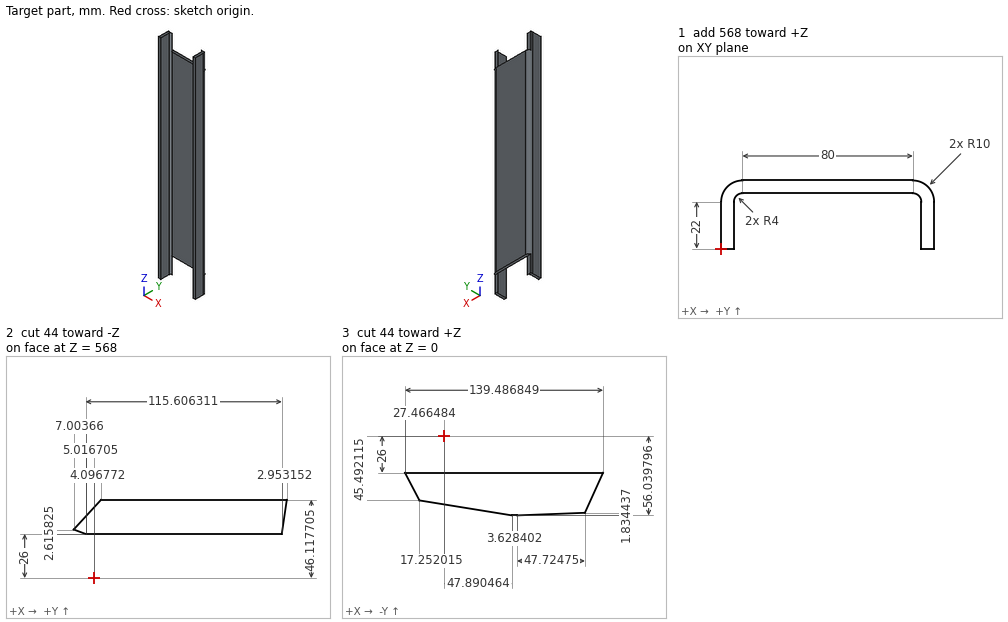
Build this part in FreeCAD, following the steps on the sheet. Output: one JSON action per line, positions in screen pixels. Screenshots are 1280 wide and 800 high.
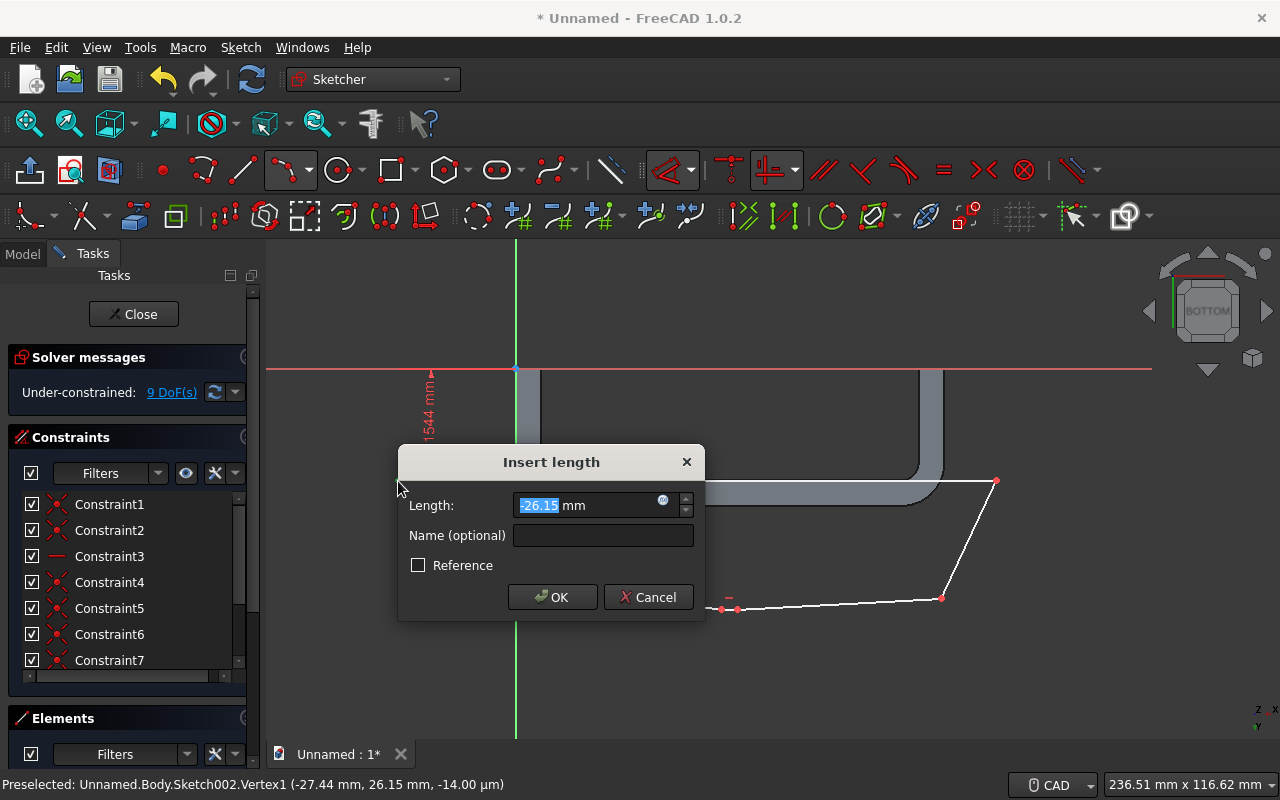
{"action": "type", "text": "-26"}
{"action": "key", "text": "Return"}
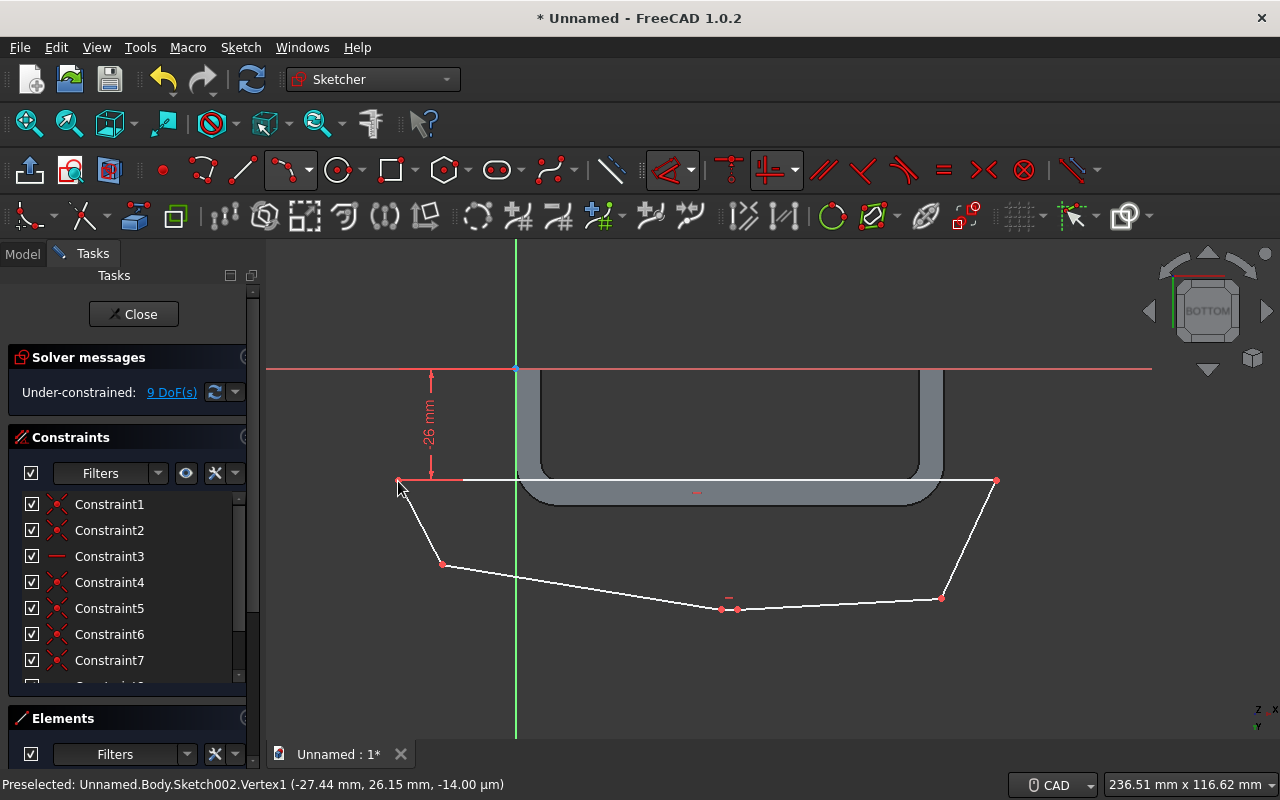
{"action": "scroll", "coordinate": [729, 610], "scroll_direction": "up", "scroll_amount": 5}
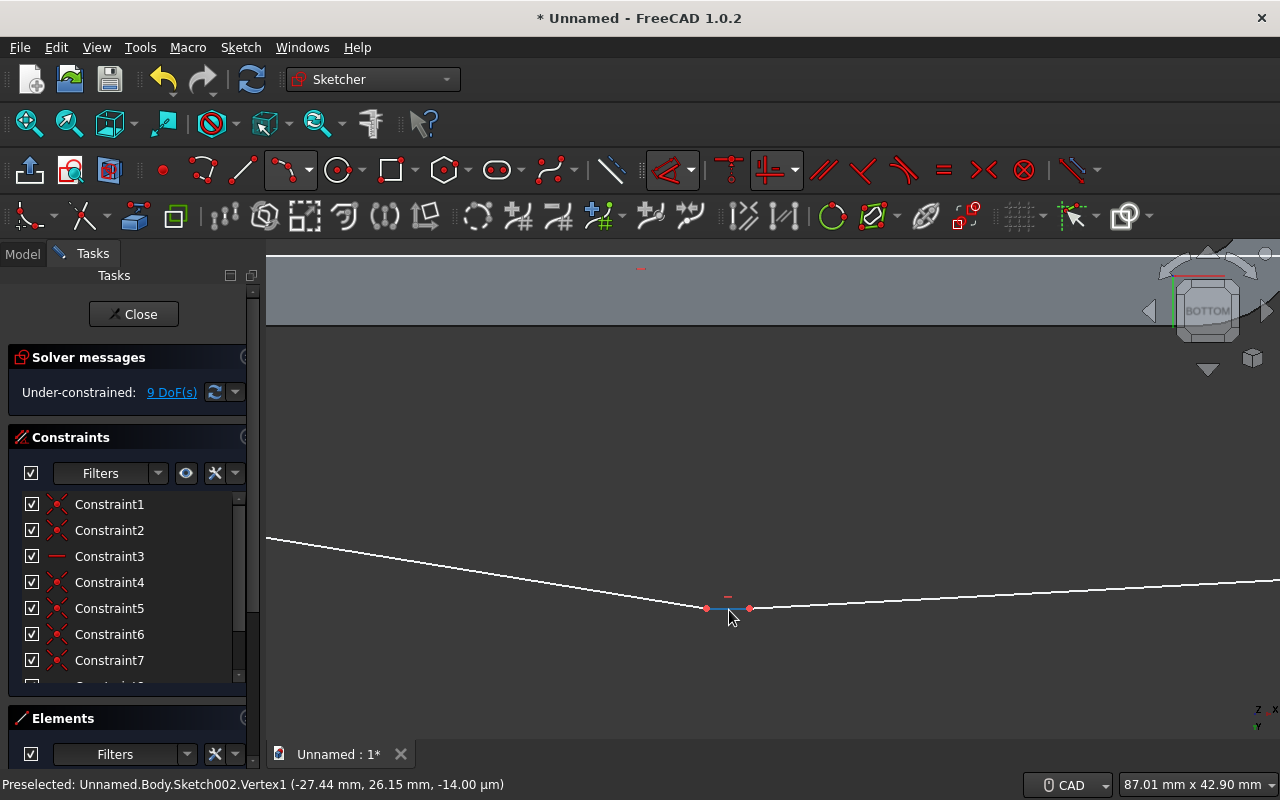
{"action": "left_click", "coordinate": [728, 609]}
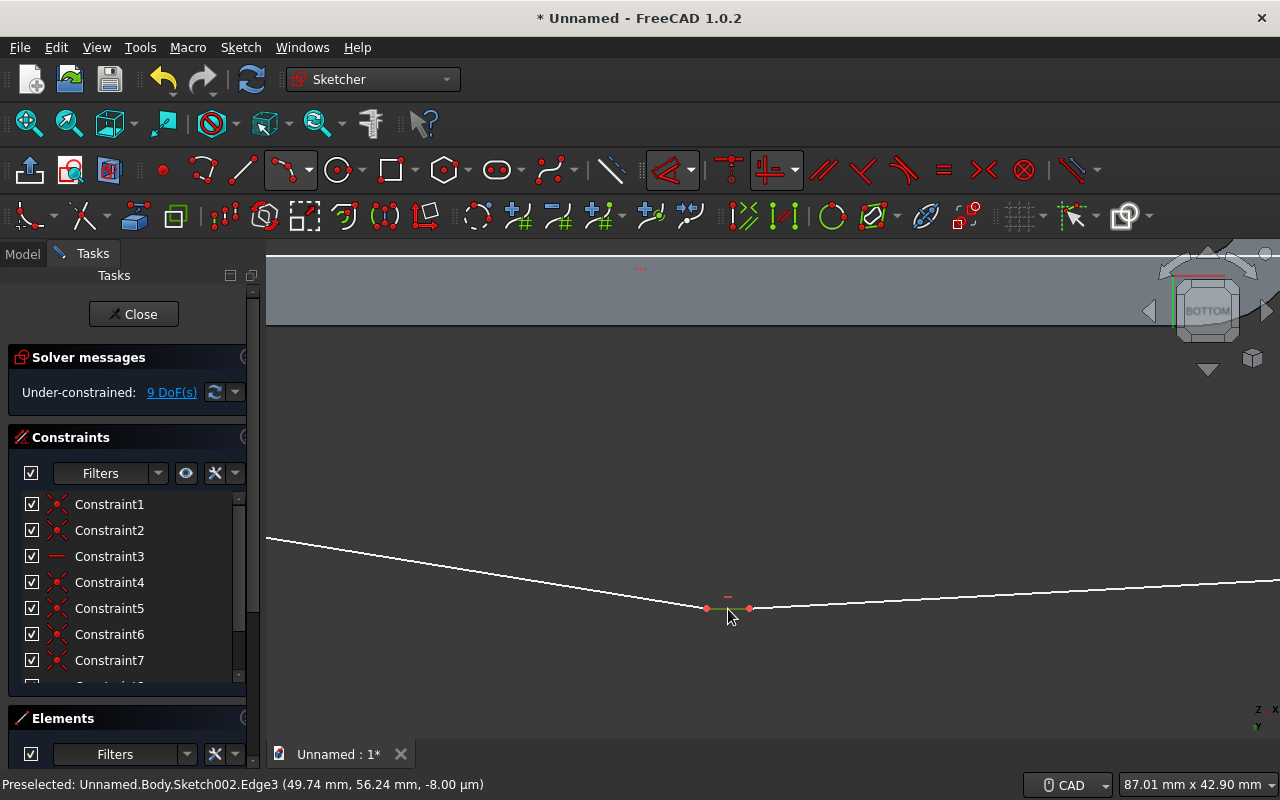
{"action": "left_click", "coordinate": [694, 170]}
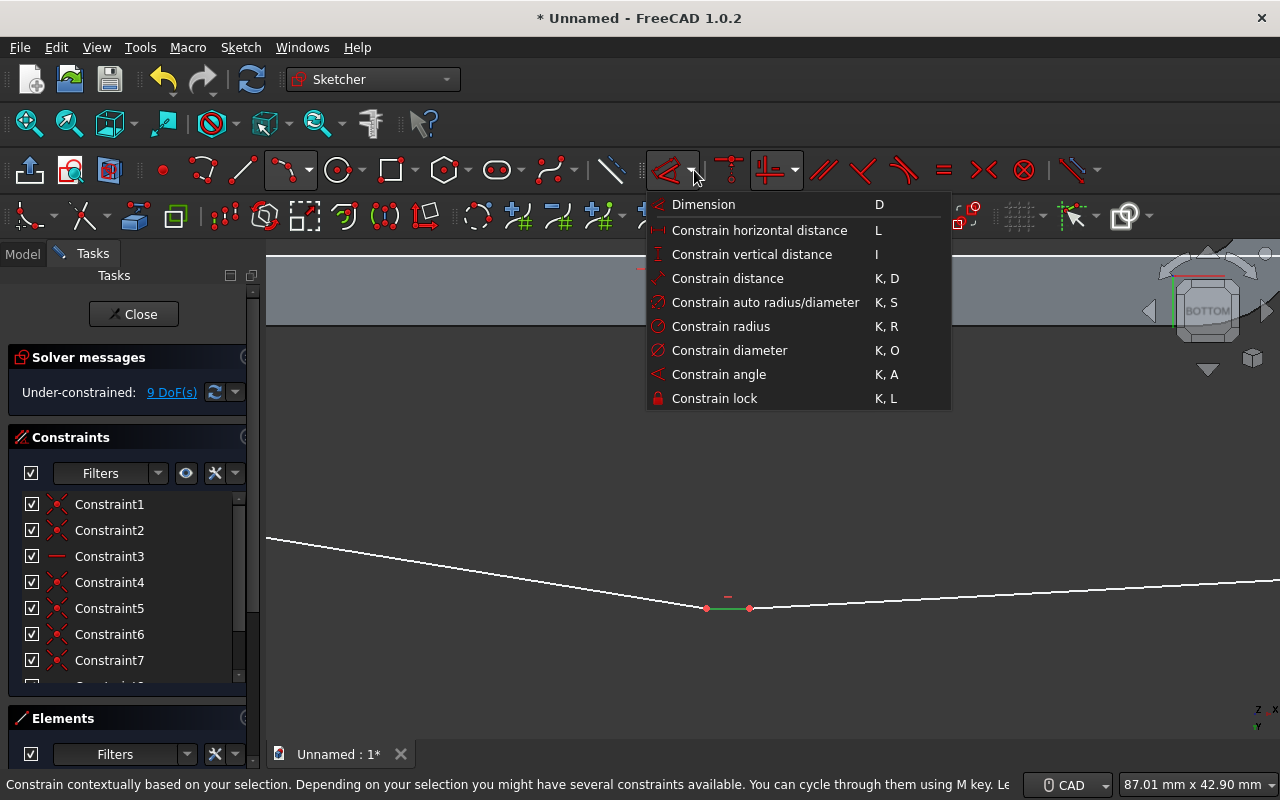
{"action": "left_click", "coordinate": [799, 230]}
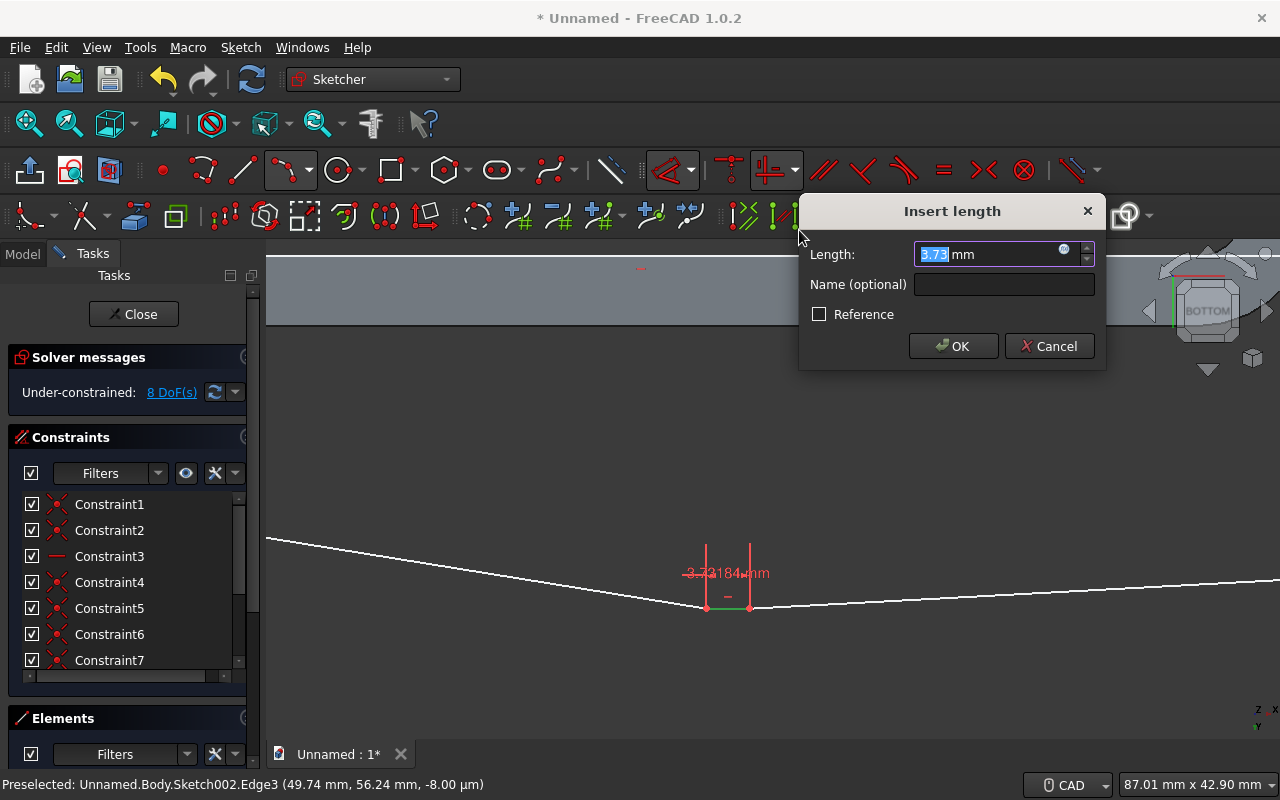
{"action": "type", "text": "3.628402"}
{"action": "key", "text": "Return"}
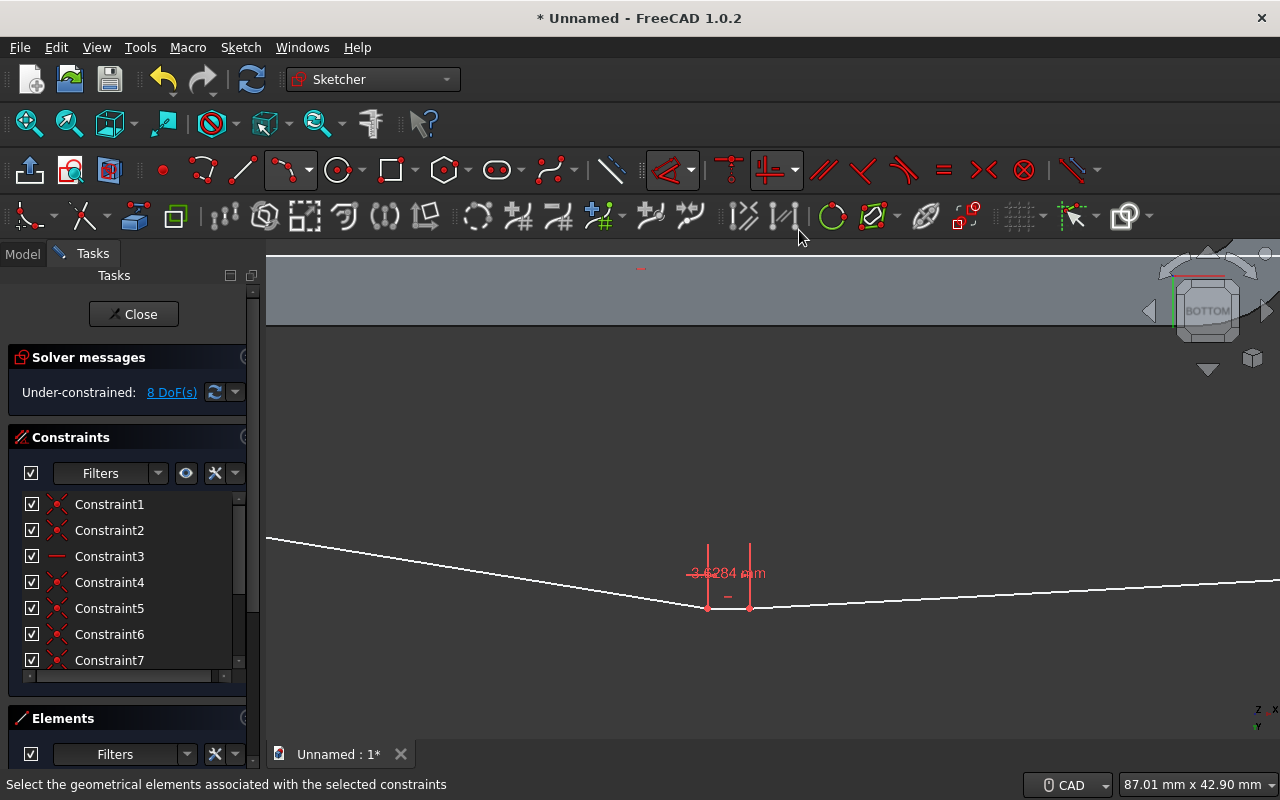
{"action": "left_click", "coordinate": [916, 600]}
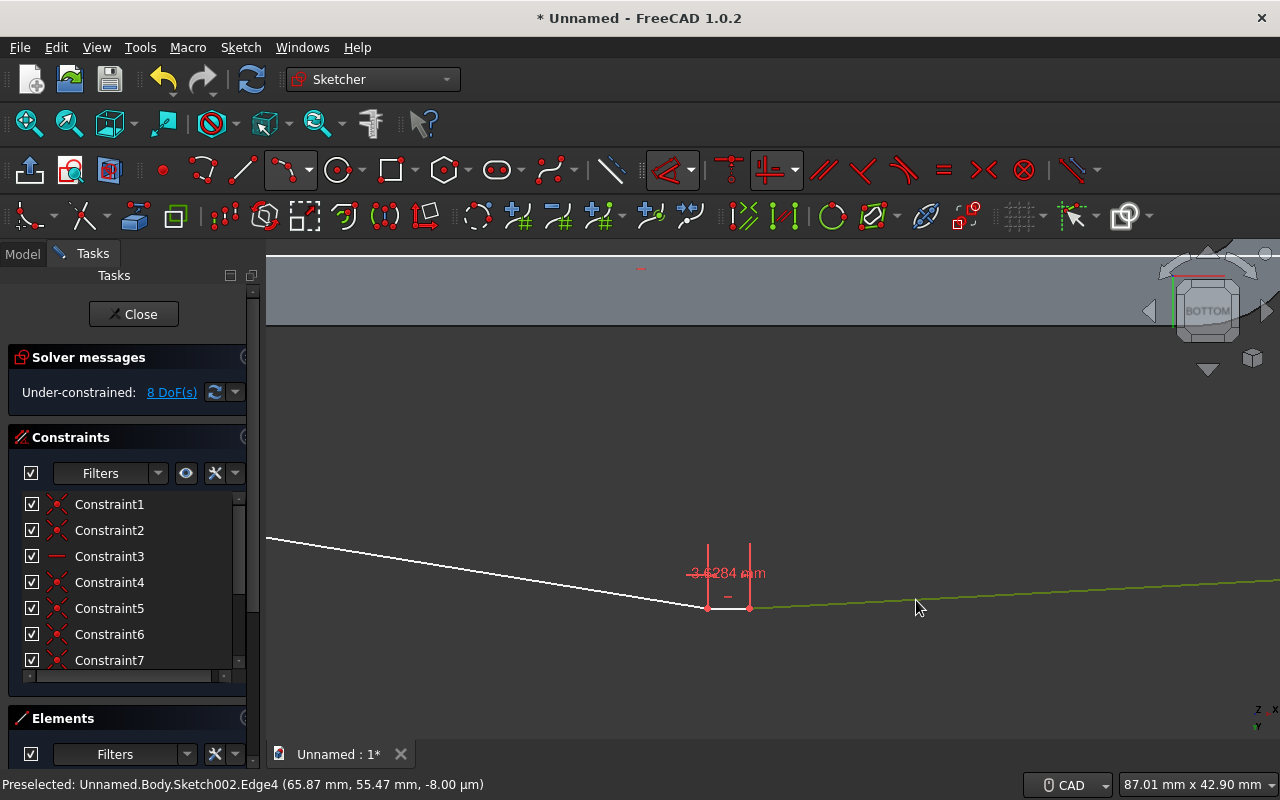
{"action": "key", "text": "l"}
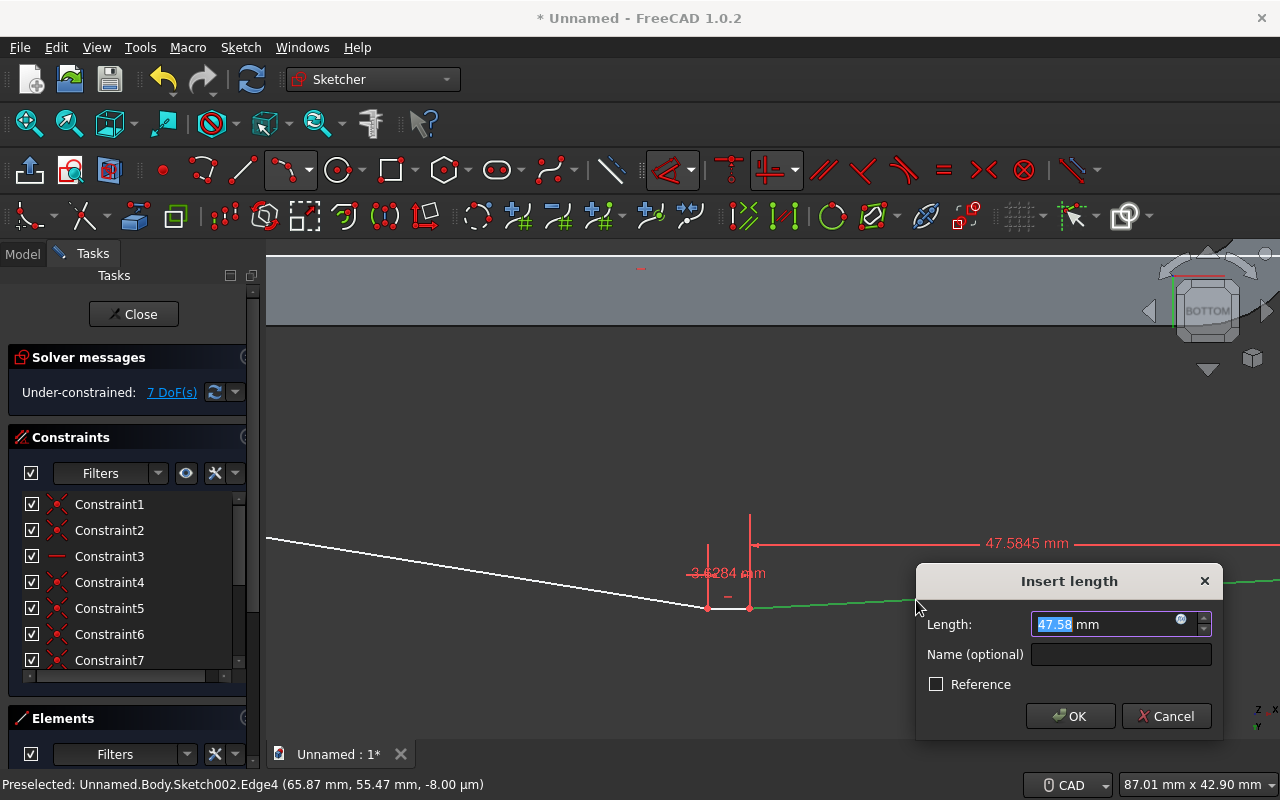
{"action": "type", "text": "47.72475"}
{"action": "key", "text": "Return"}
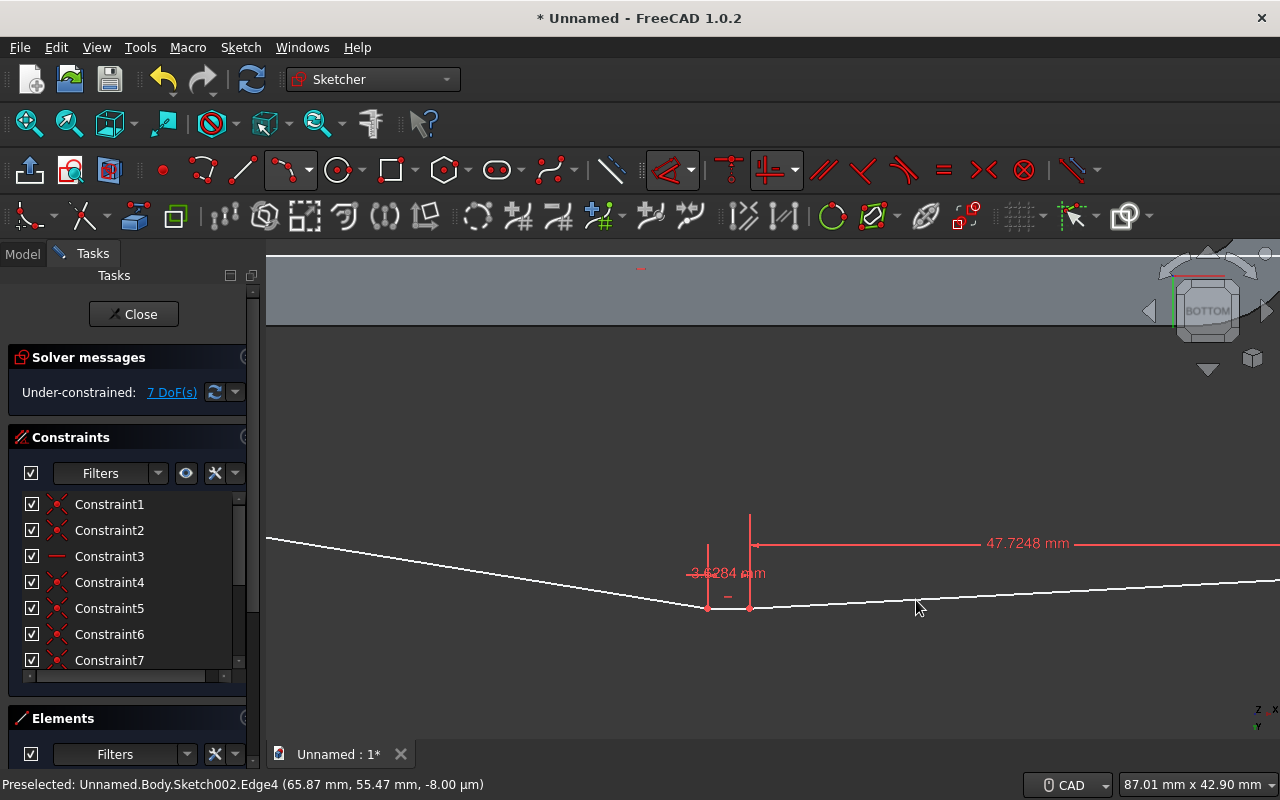
{"action": "scroll", "coordinate": [917, 600], "scroll_direction": "up", "scroll_amount": 4}